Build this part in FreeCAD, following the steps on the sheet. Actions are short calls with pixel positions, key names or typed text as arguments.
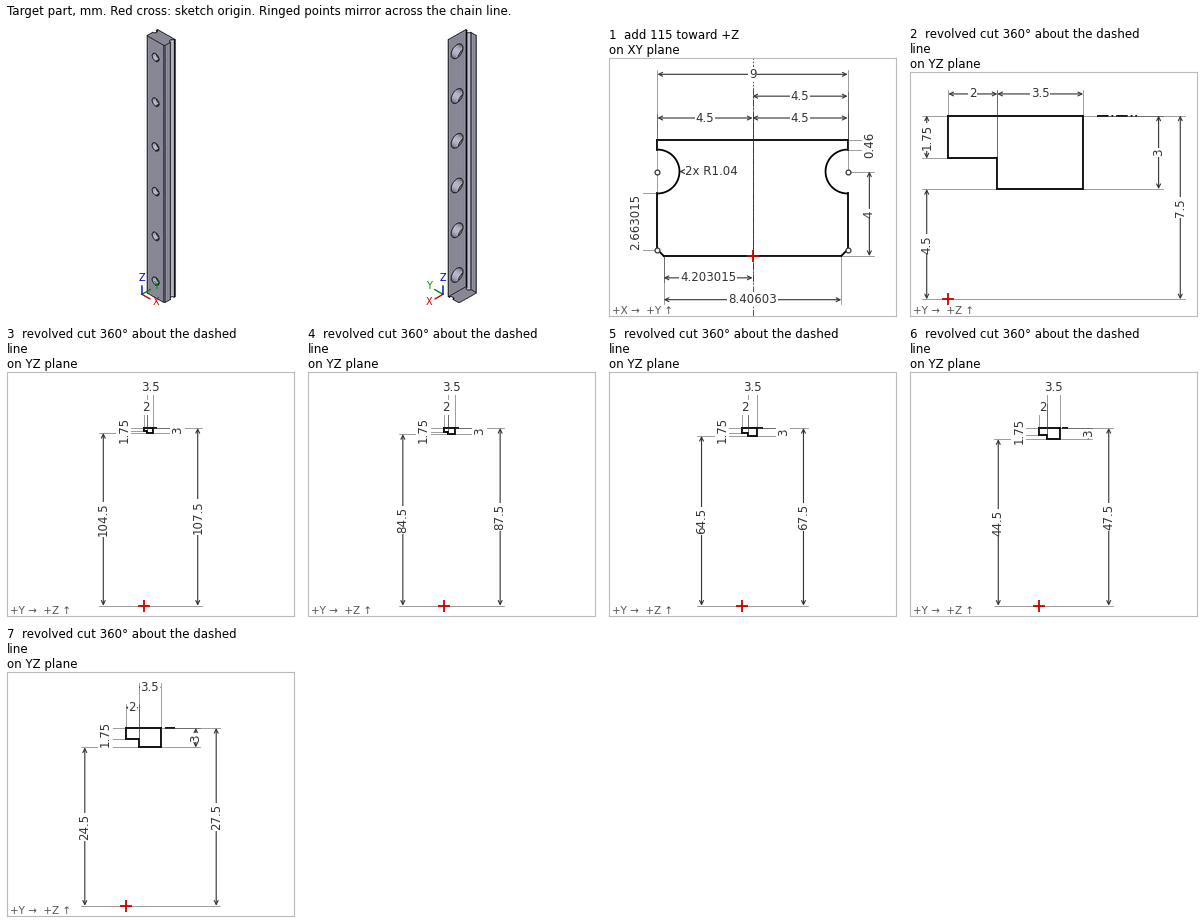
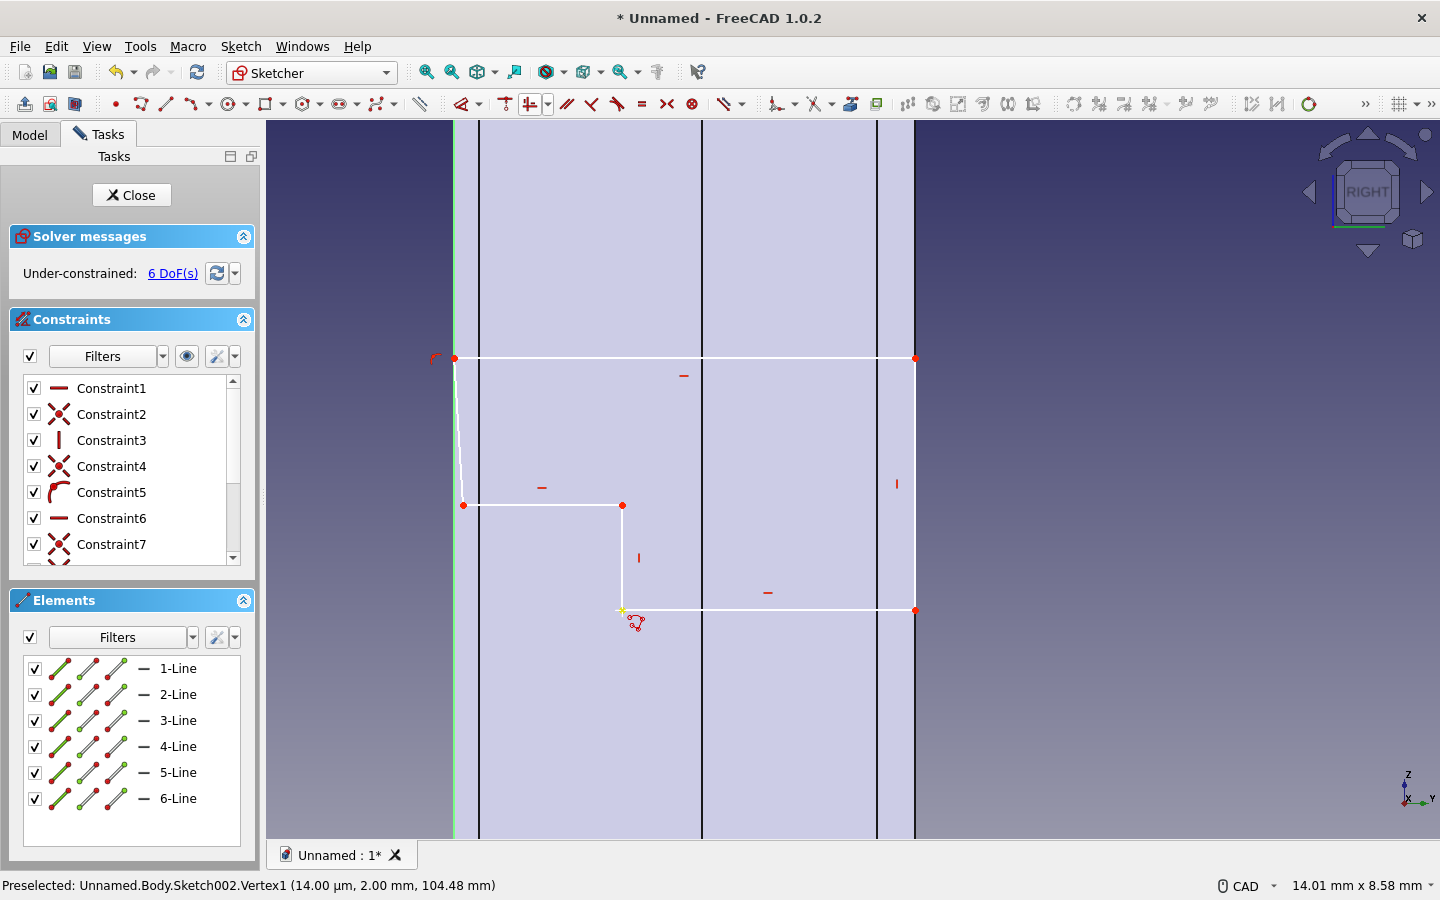
key(g)
key(l)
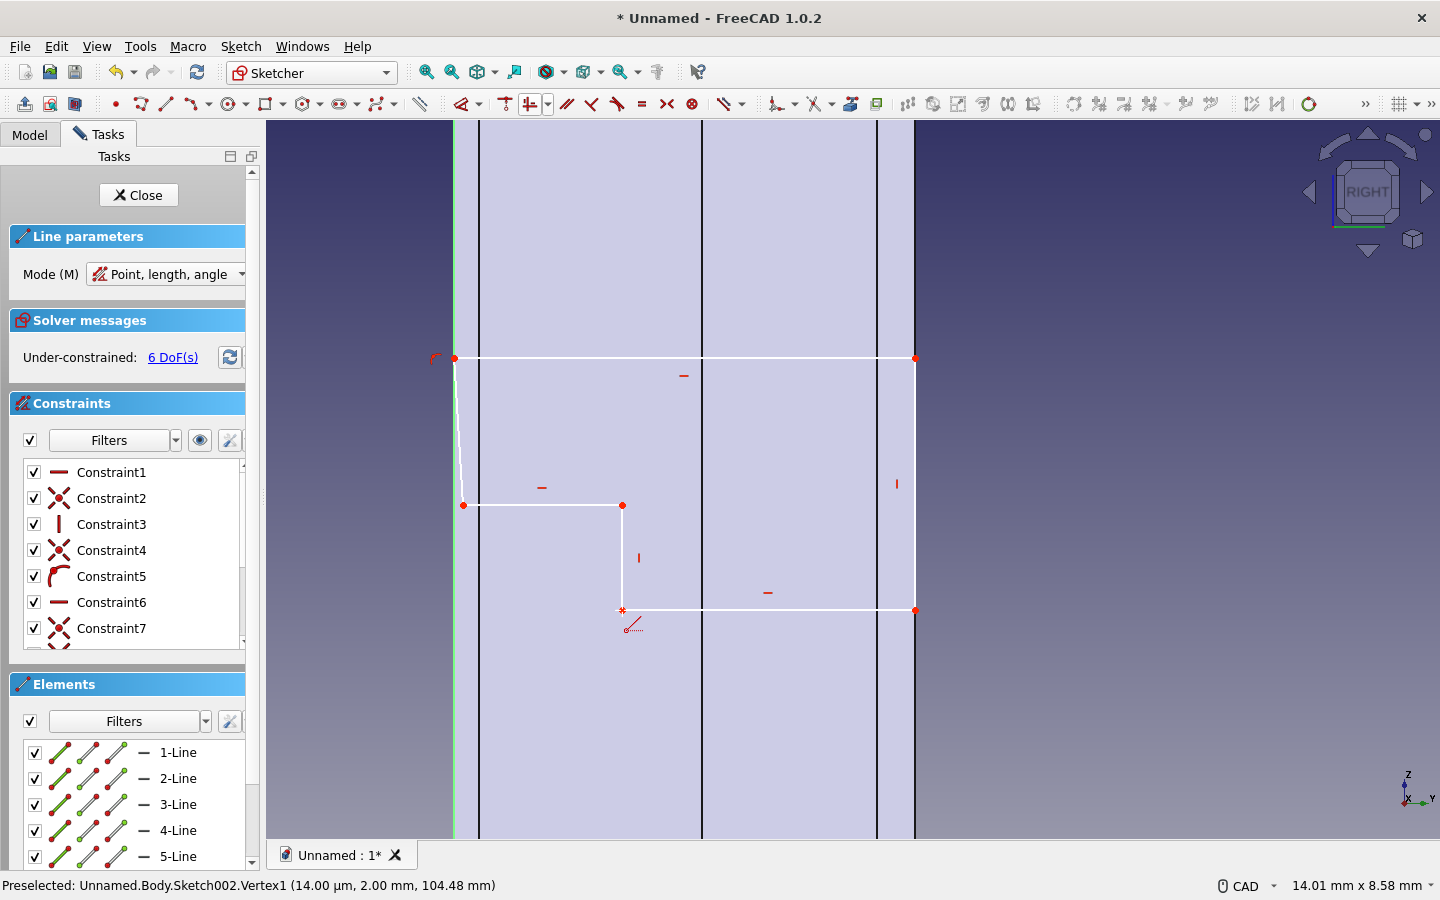
click(961, 357)
click(1100, 357)
key(Escape)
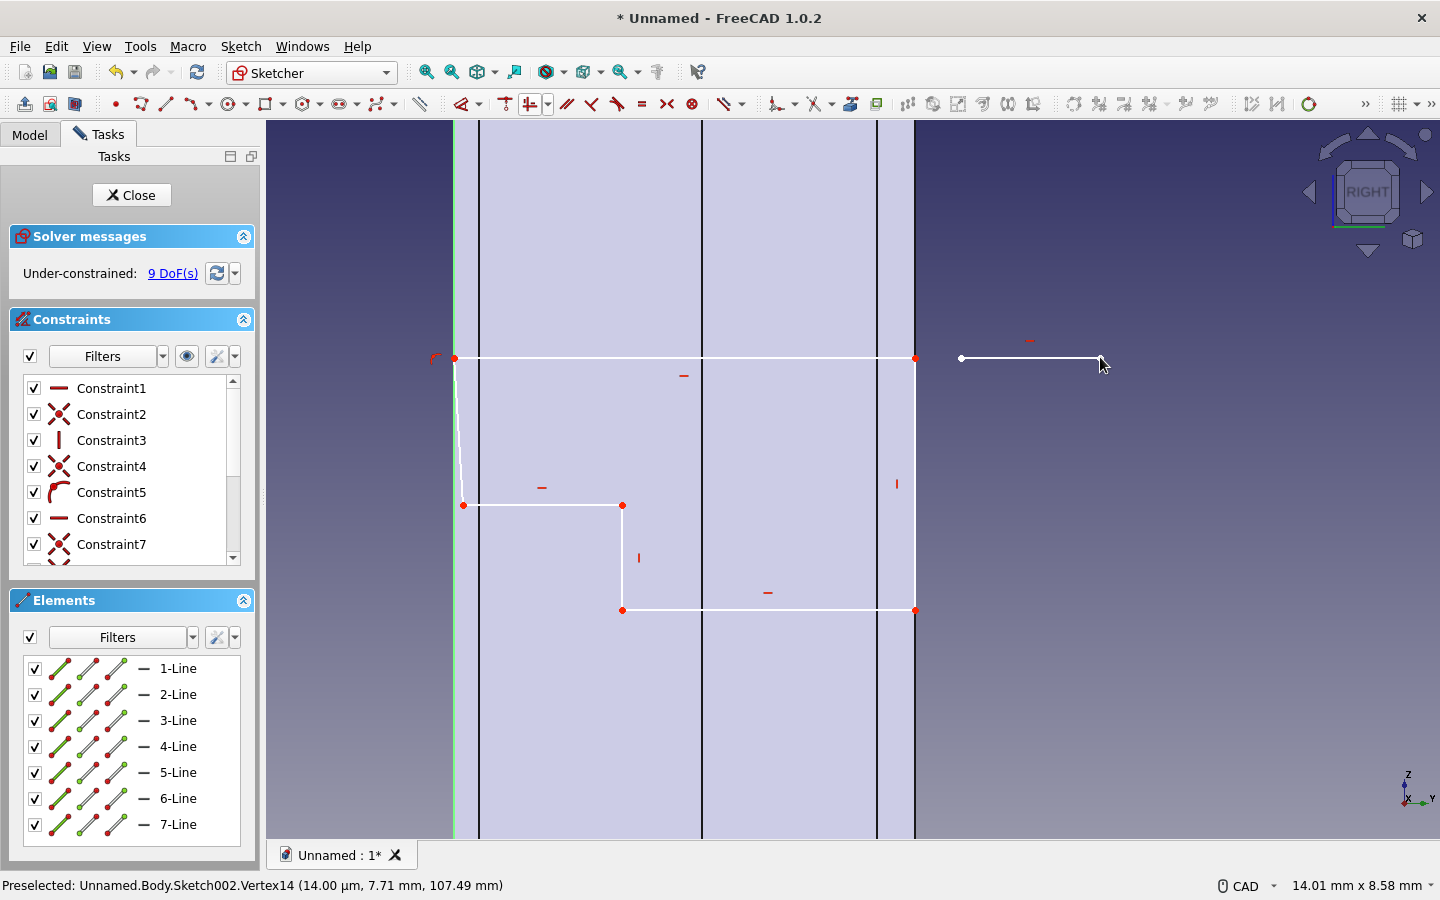
click(1003, 358)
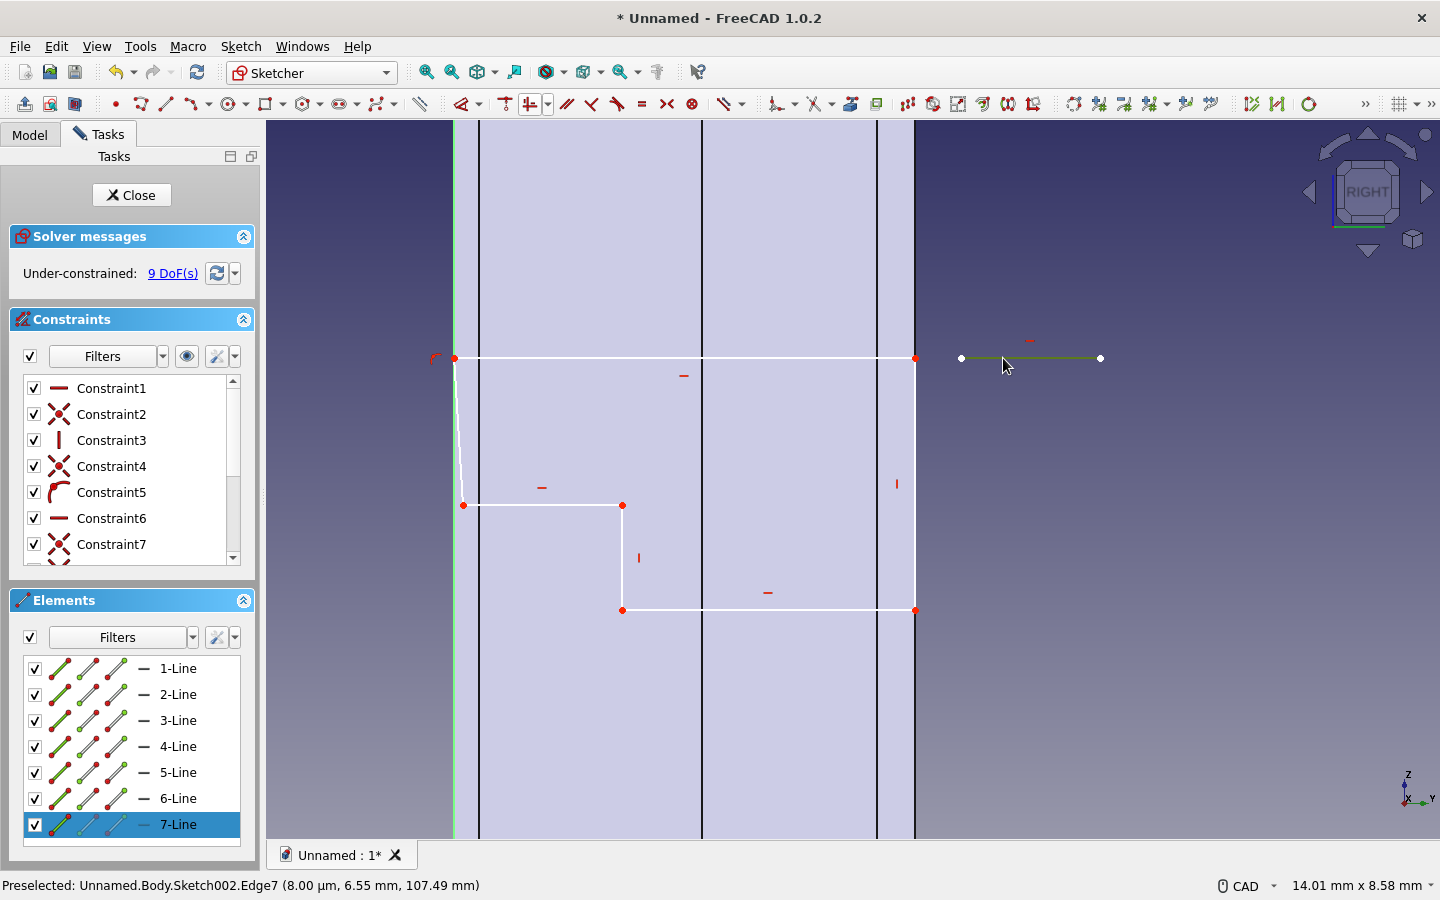
key(g)
key(n)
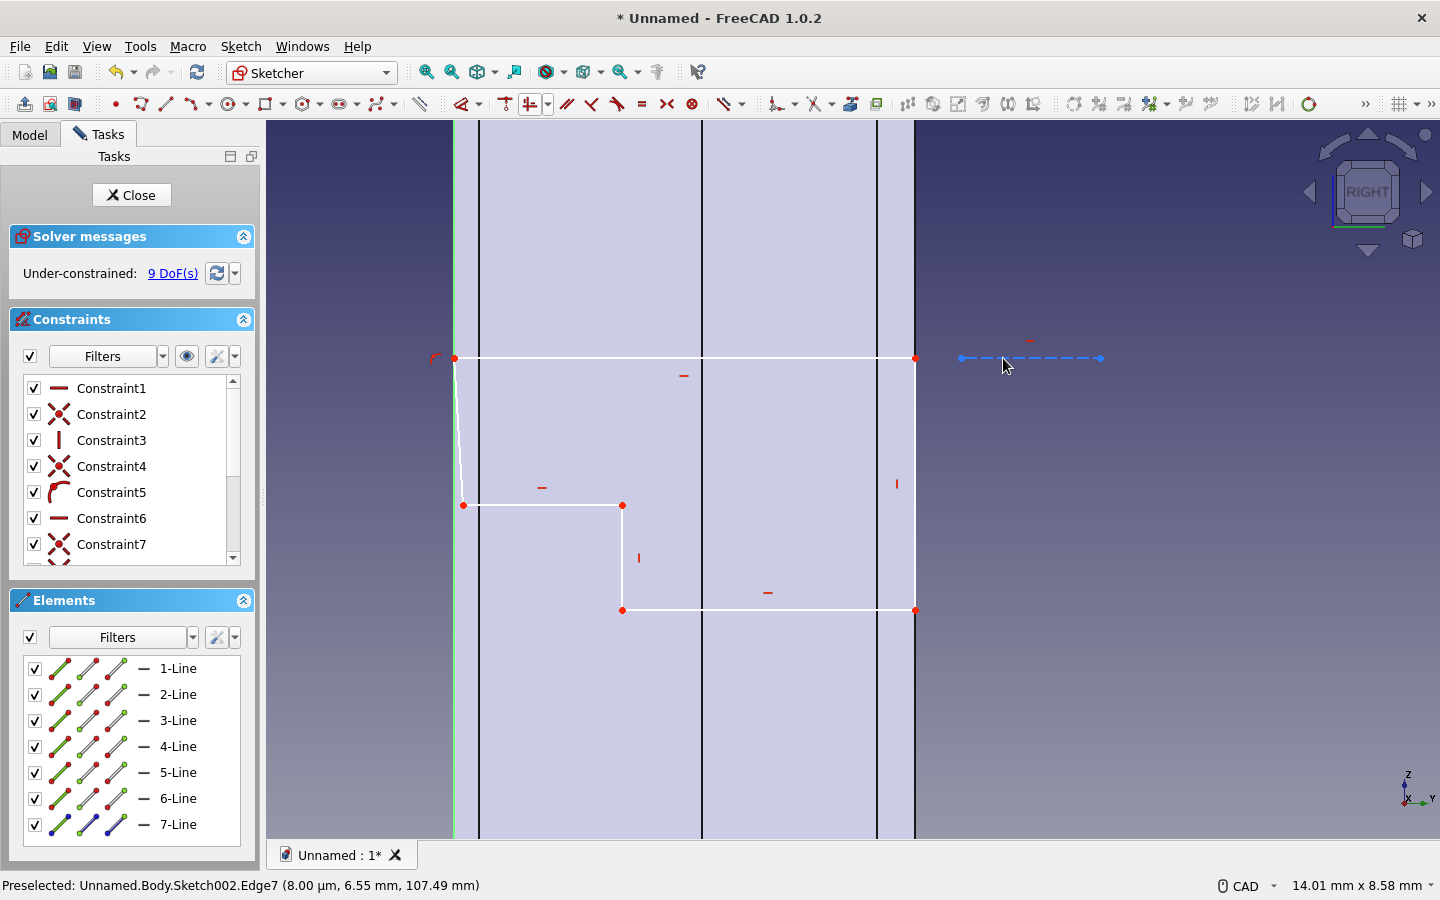
click(457, 402)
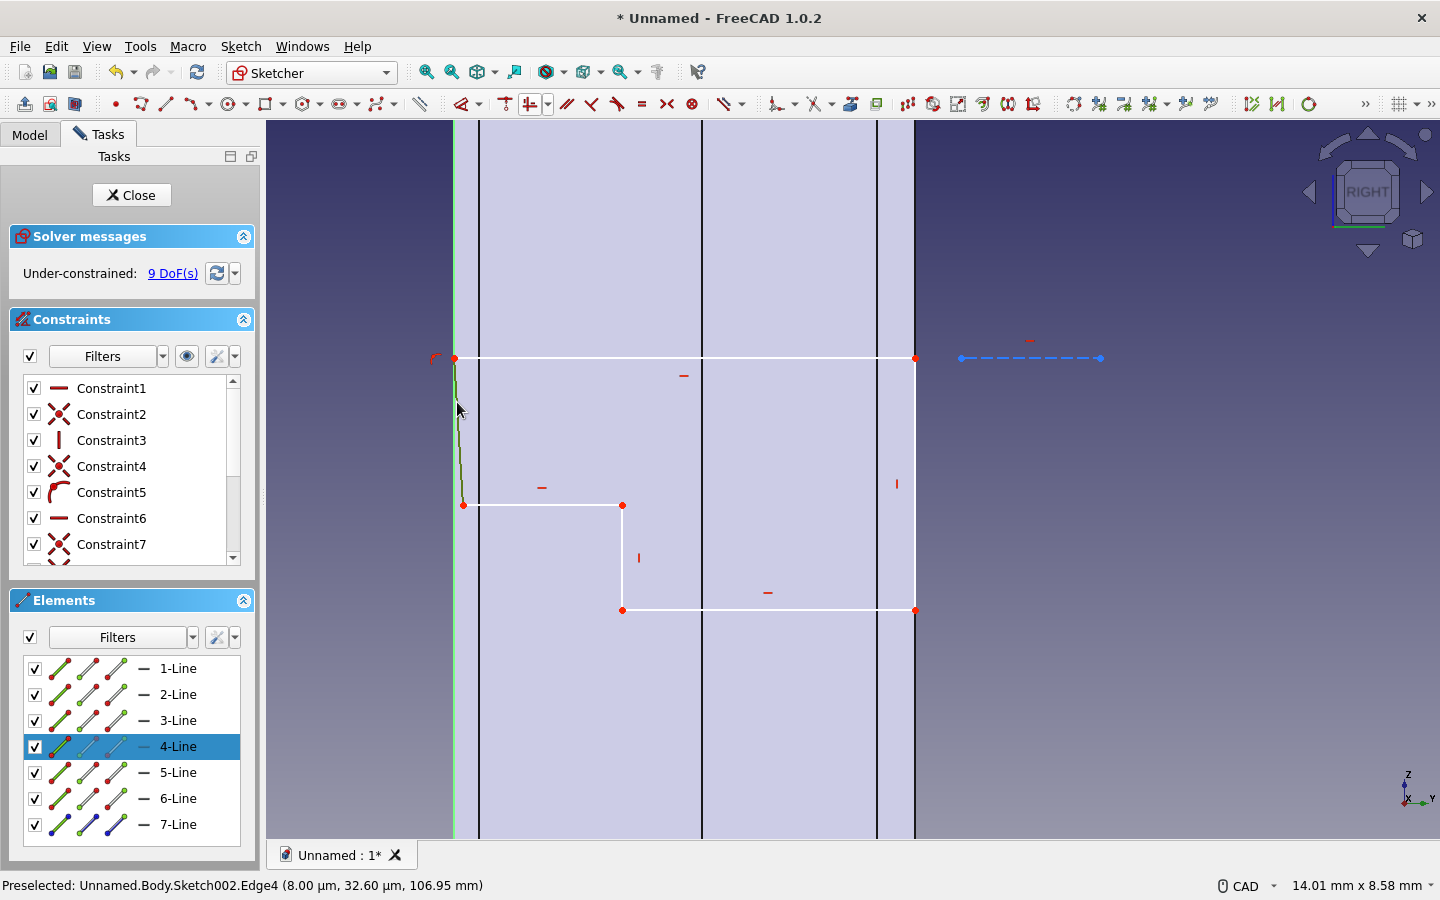
key(v)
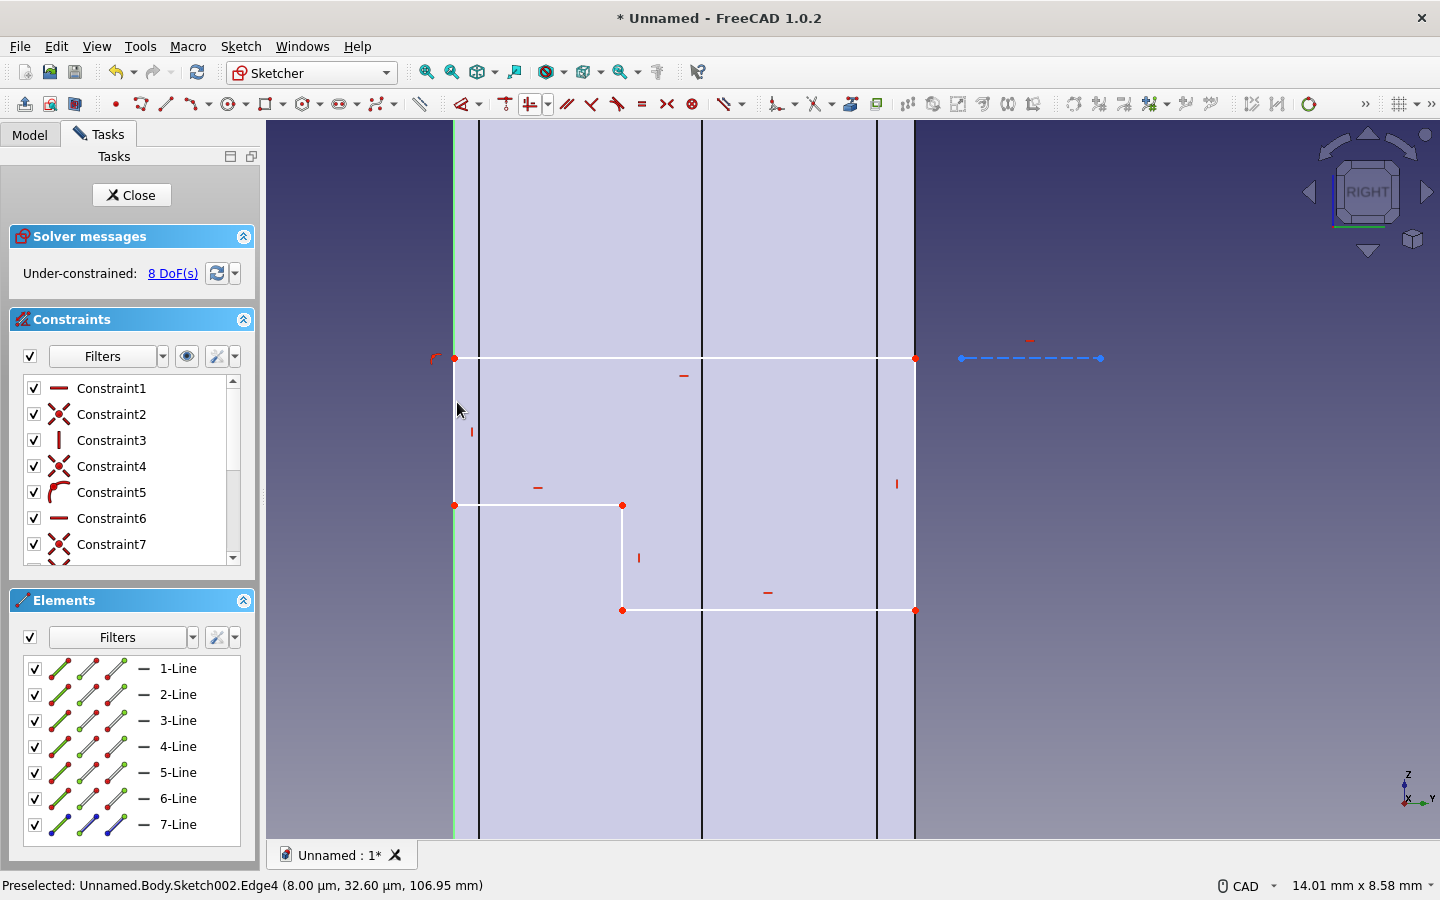
key(d)